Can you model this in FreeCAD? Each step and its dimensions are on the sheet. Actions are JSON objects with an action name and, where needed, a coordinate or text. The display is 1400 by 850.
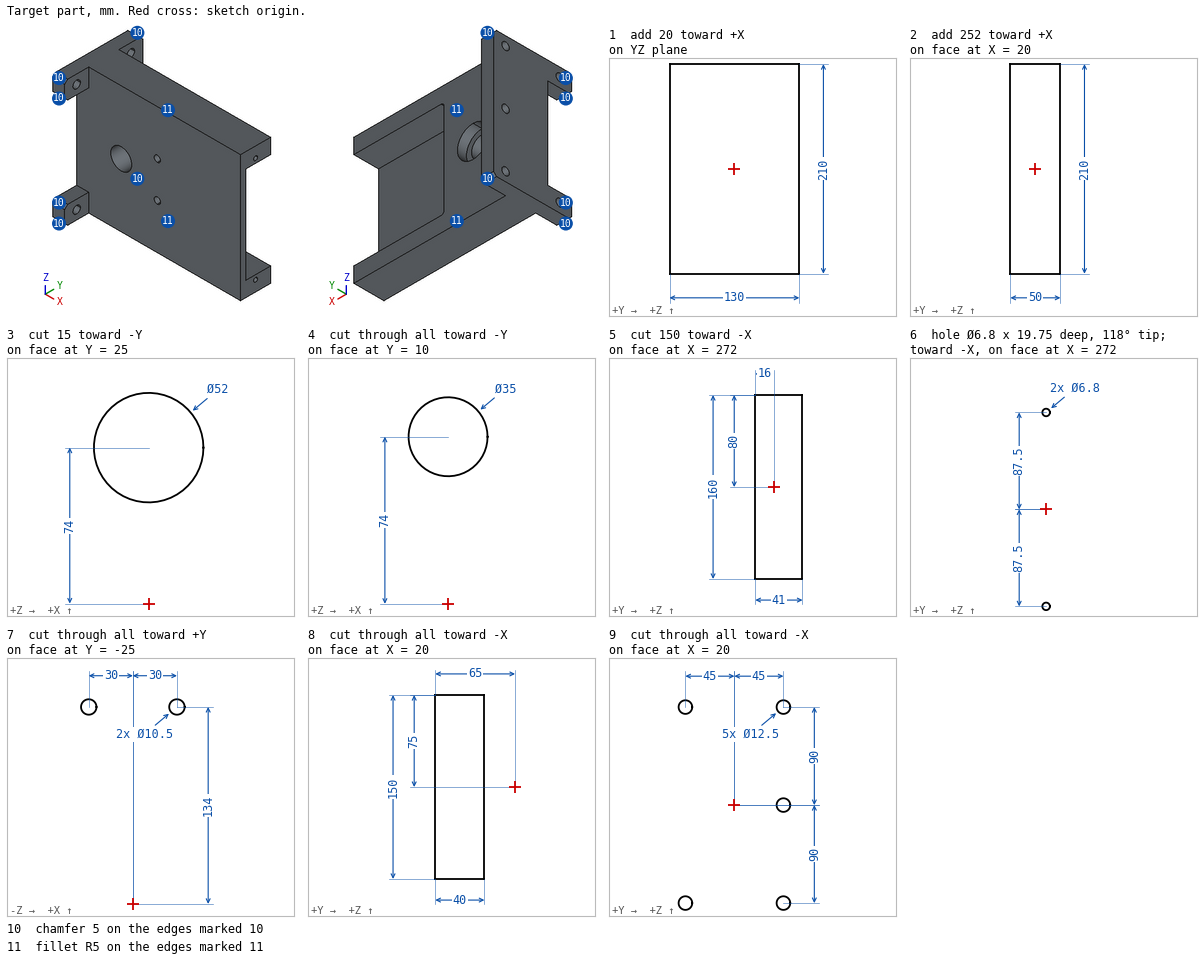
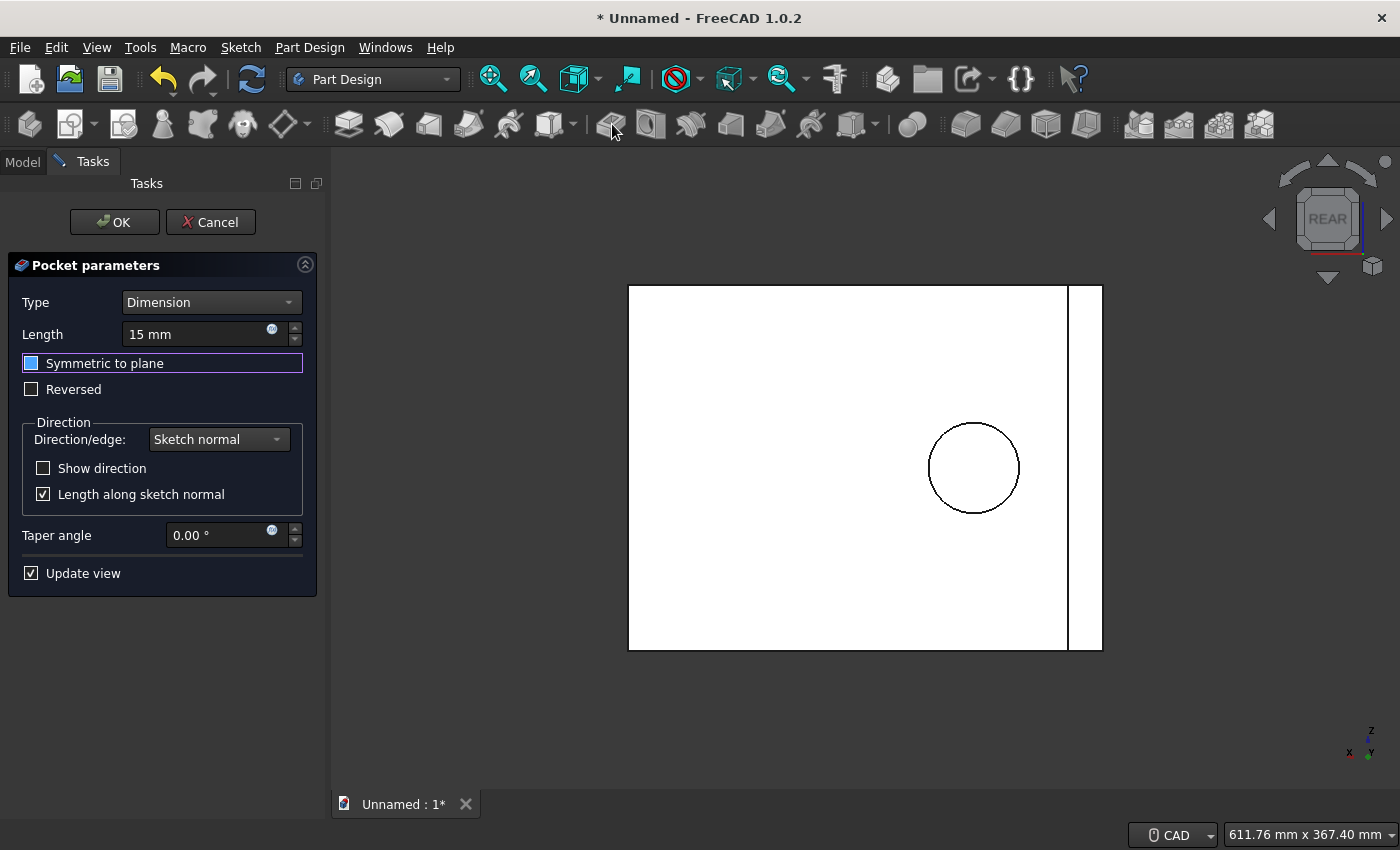
{"action": "left_click", "coordinate": [115, 222]}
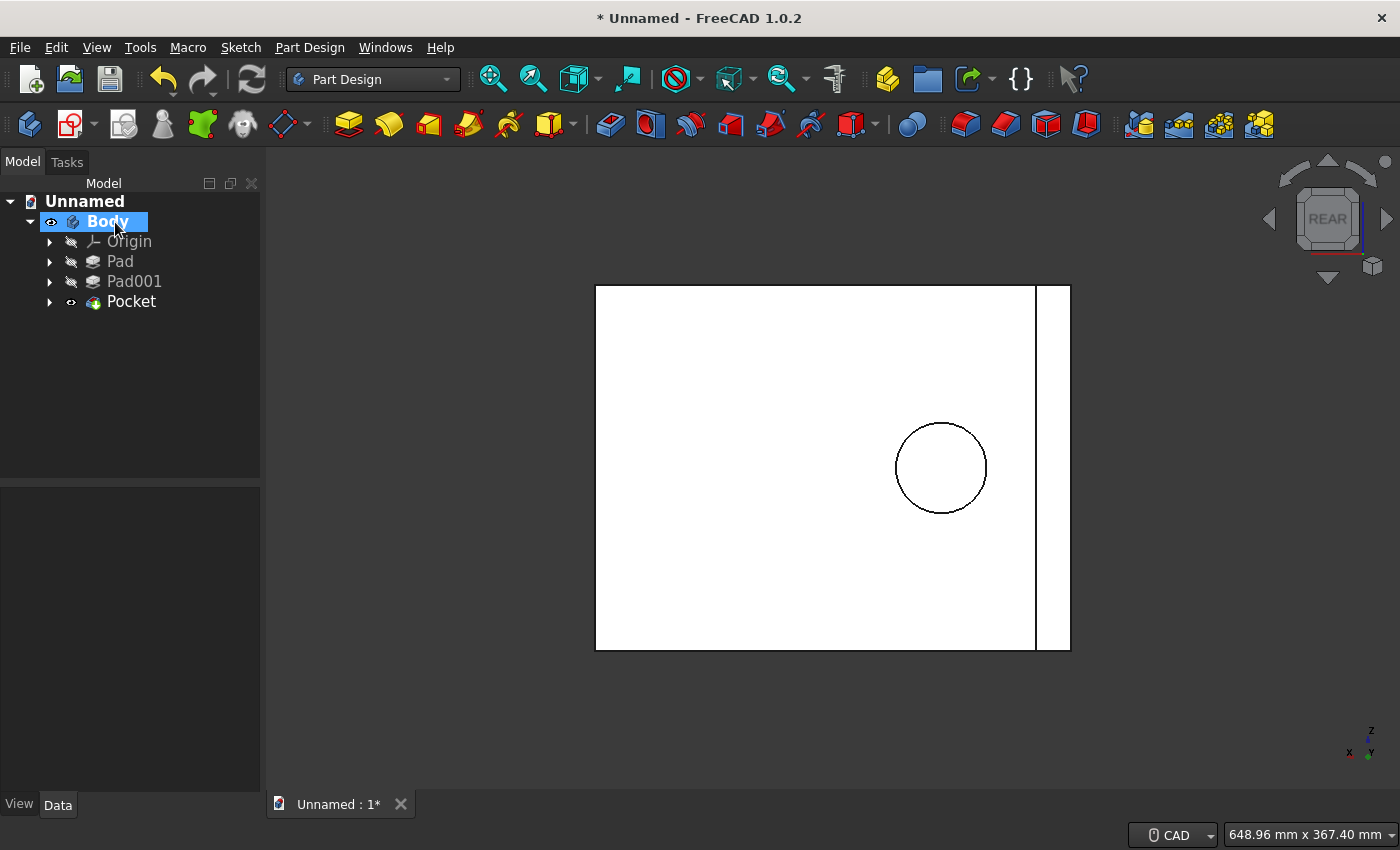
{"action": "left_click", "coordinate": [941, 467]}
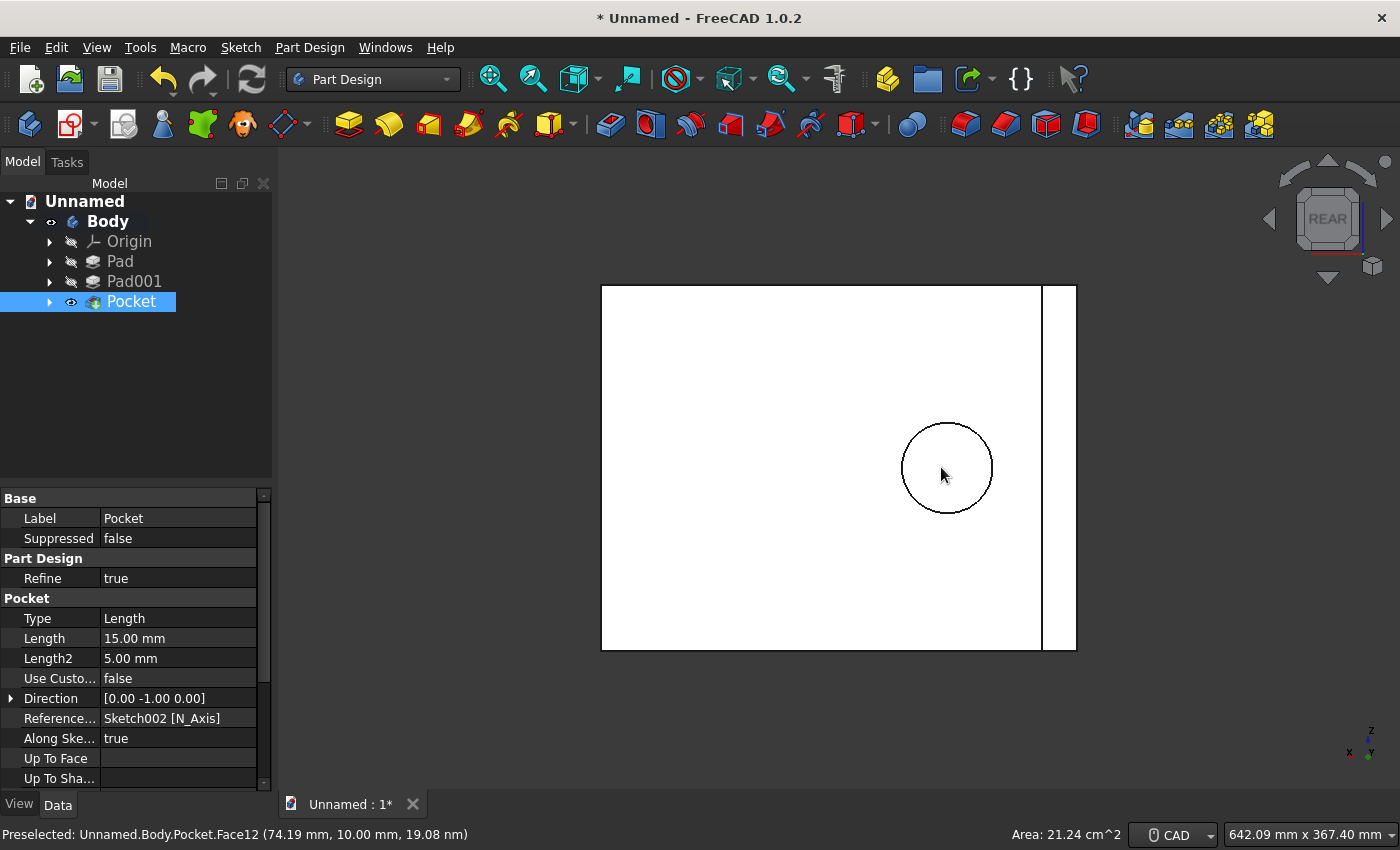
{"action": "left_click", "coordinate": [70, 124]}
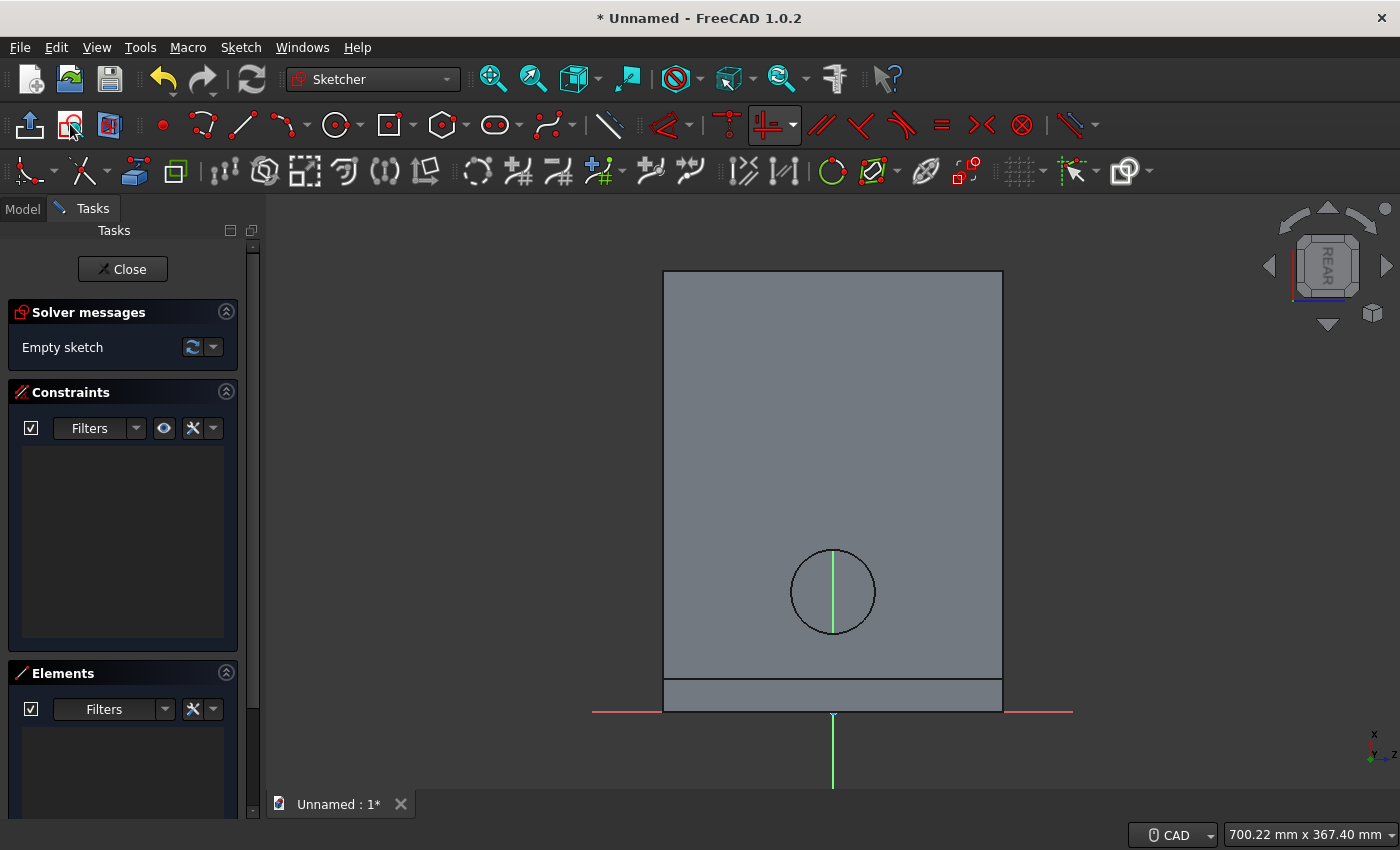
{"action": "scroll", "coordinate": [844, 608], "scroll_direction": "up", "scroll_amount": 10}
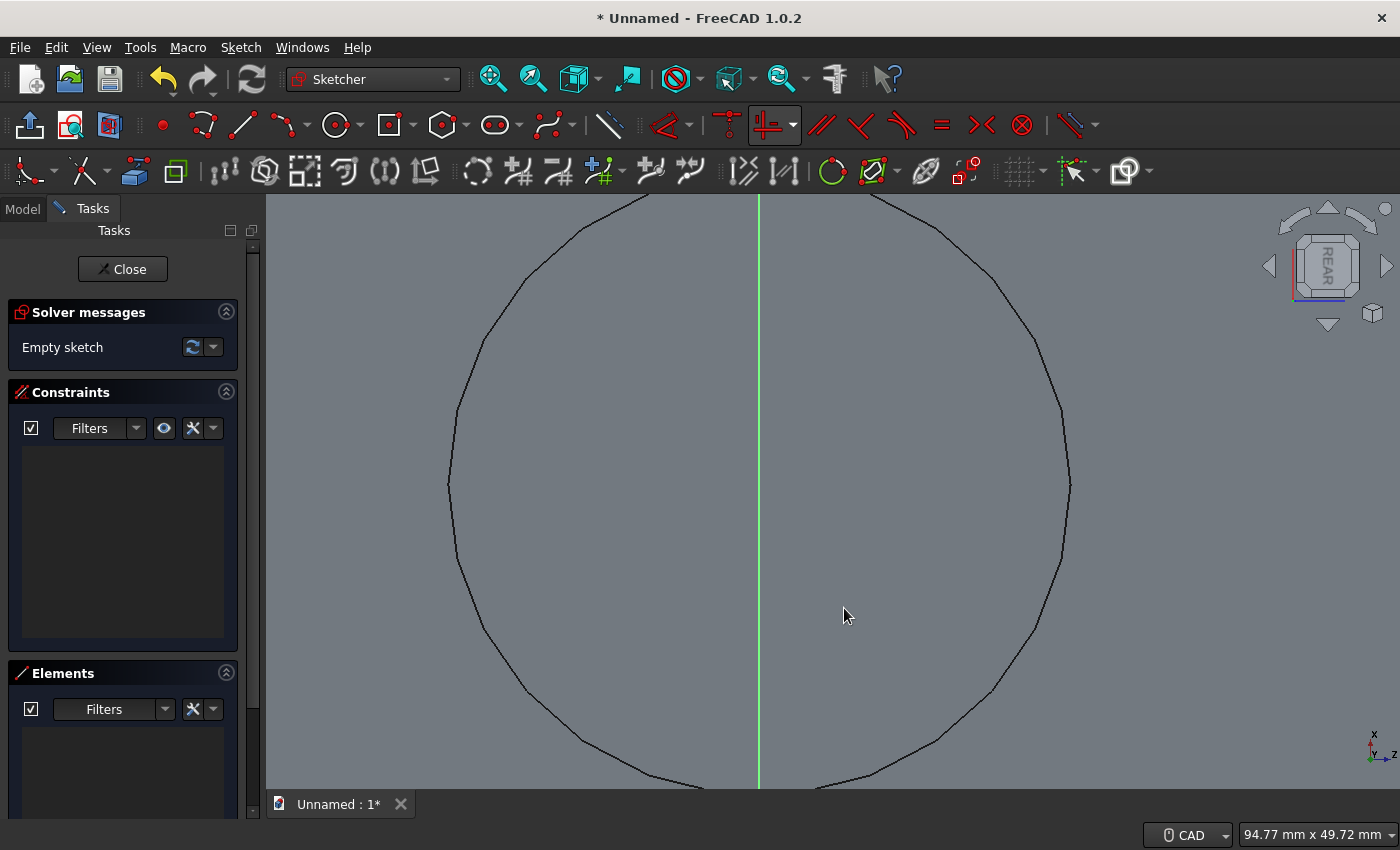
{"action": "left_click", "coordinate": [336, 126]}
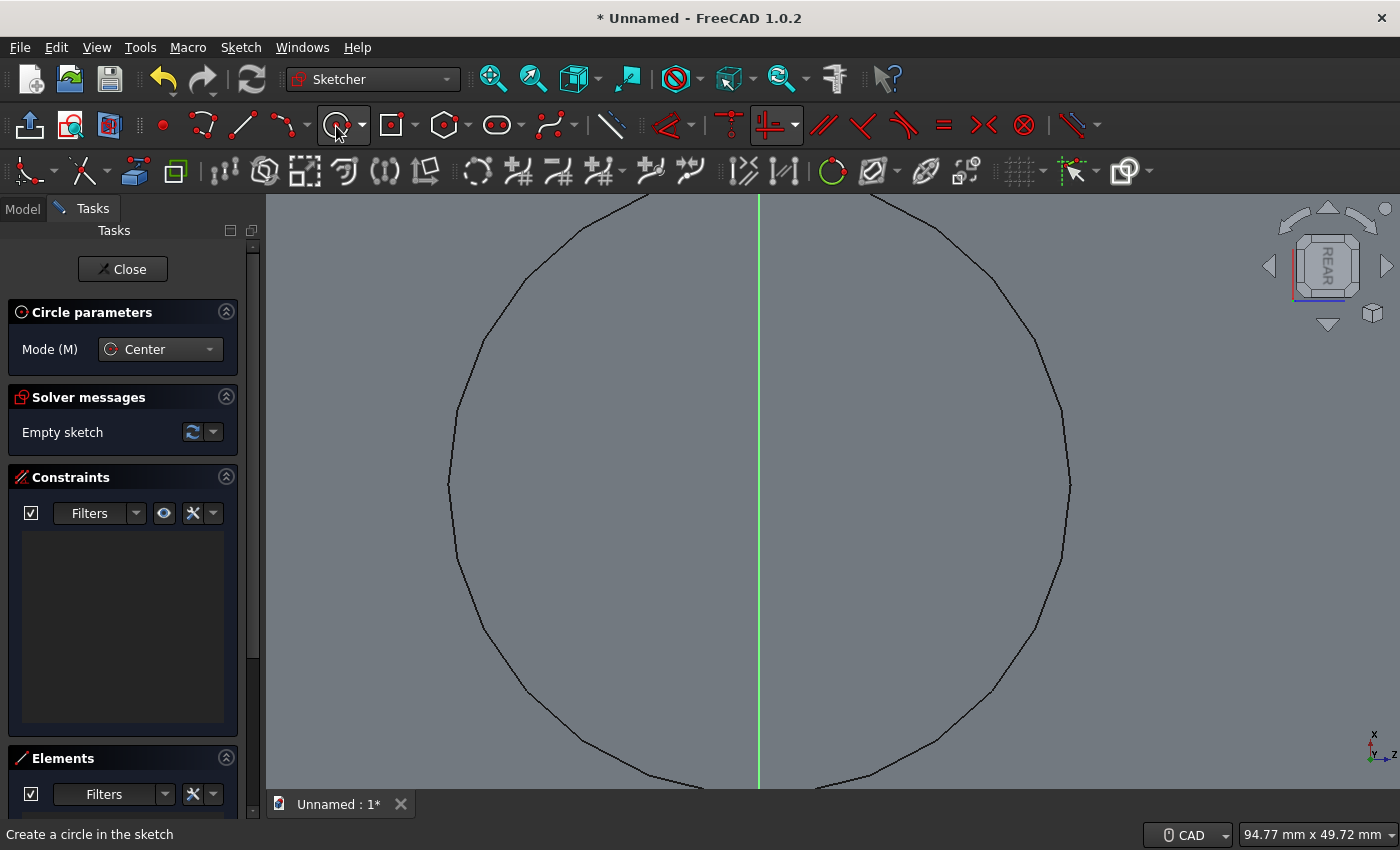
{"action": "left_click", "coordinate": [759, 485]}
{"action": "left_click", "coordinate": [908, 337]}
{"action": "key", "text": "Escape"}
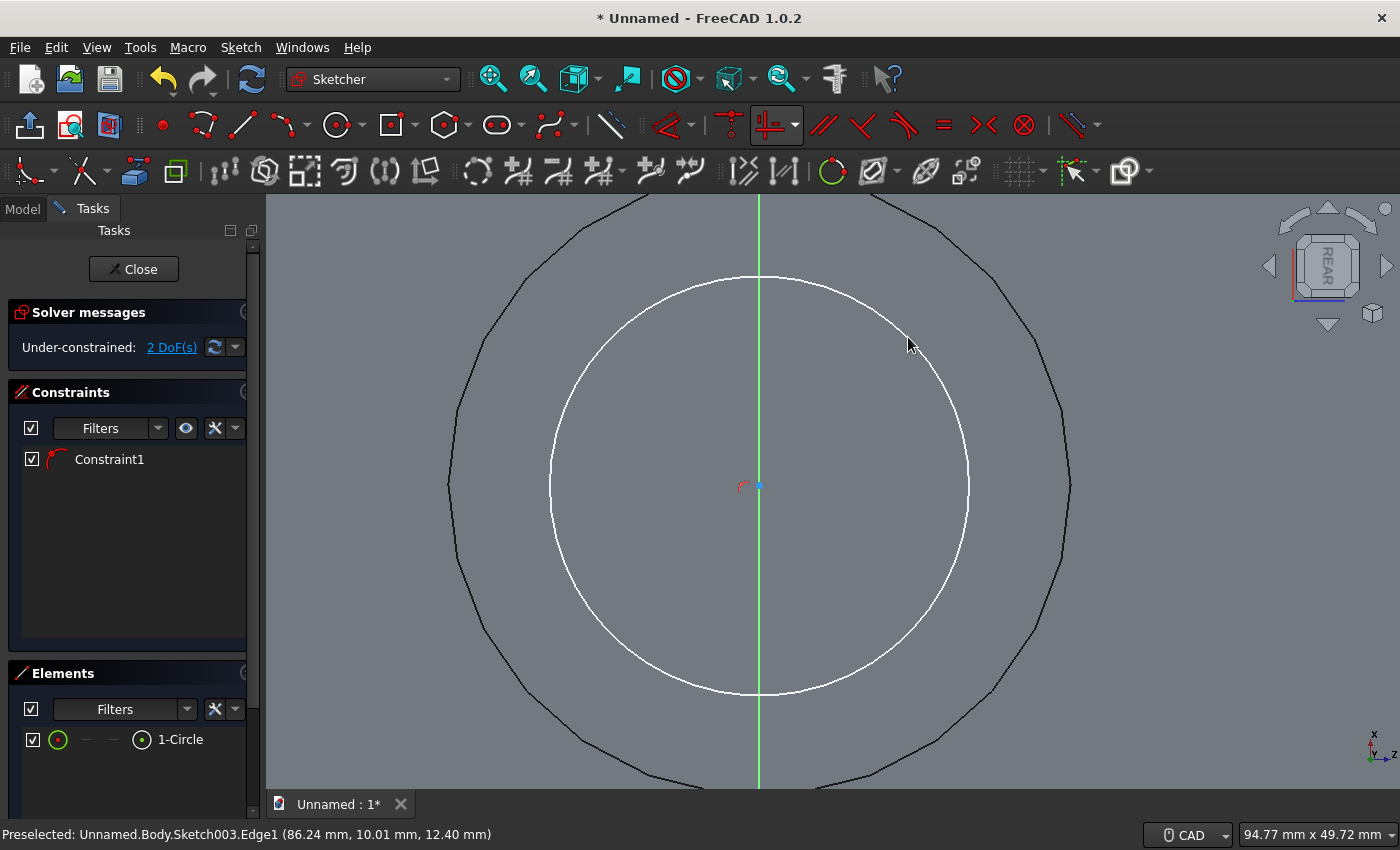
{"action": "left_click", "coordinate": [666, 126]}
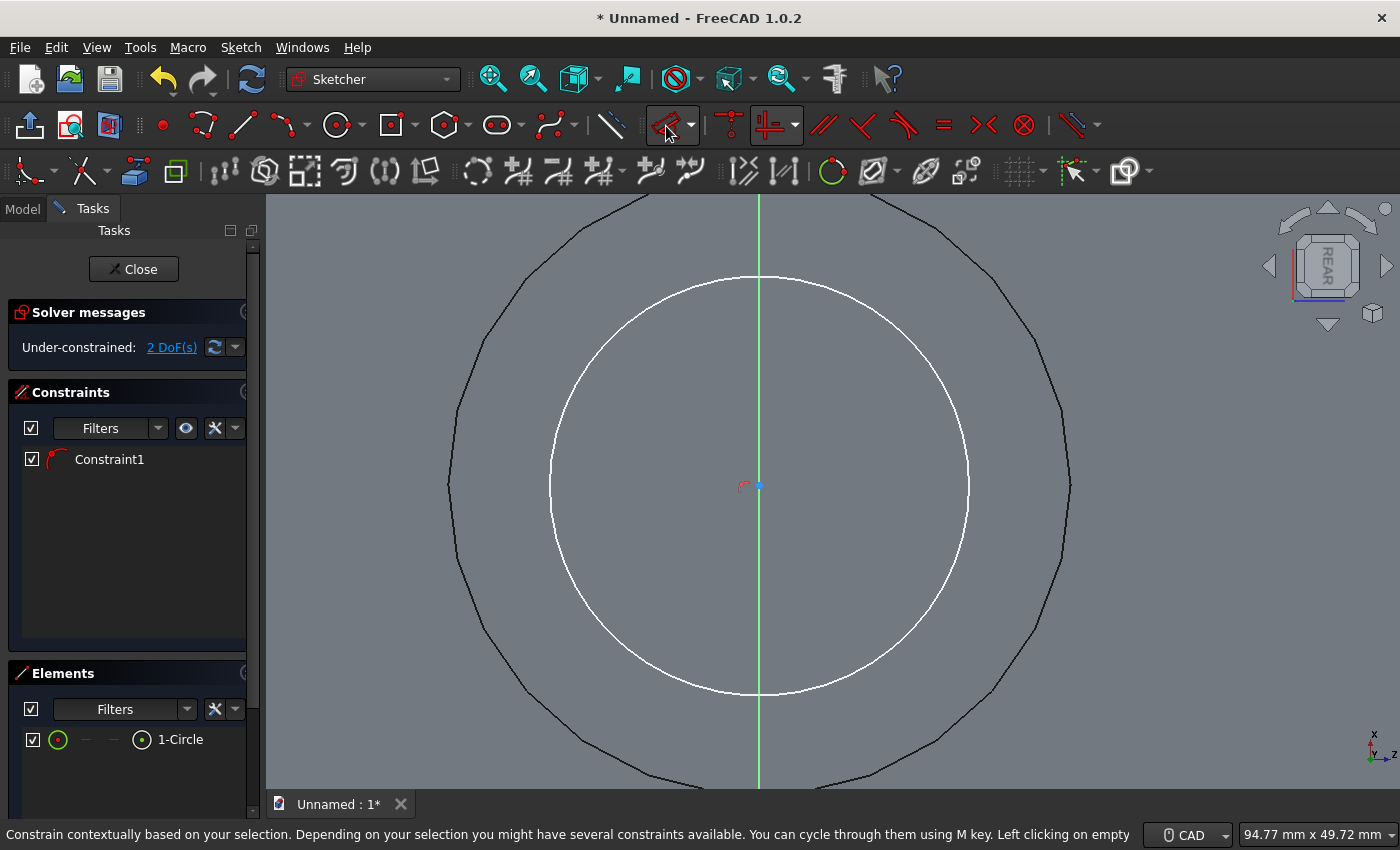
{"action": "left_click", "coordinate": [907, 337]}
{"action": "left_click", "coordinate": [930, 314]}